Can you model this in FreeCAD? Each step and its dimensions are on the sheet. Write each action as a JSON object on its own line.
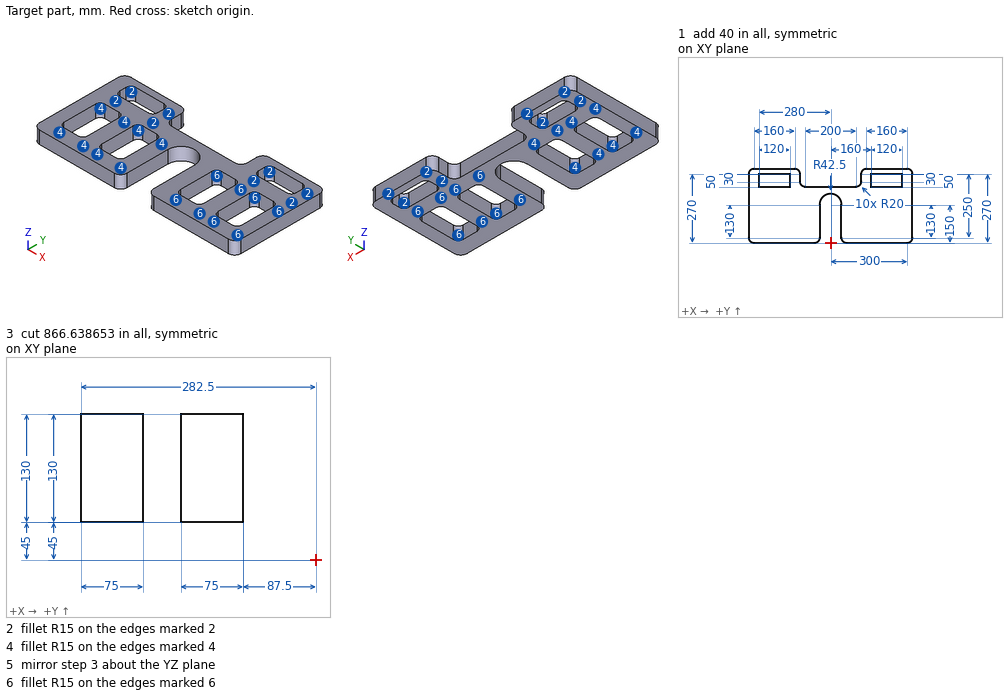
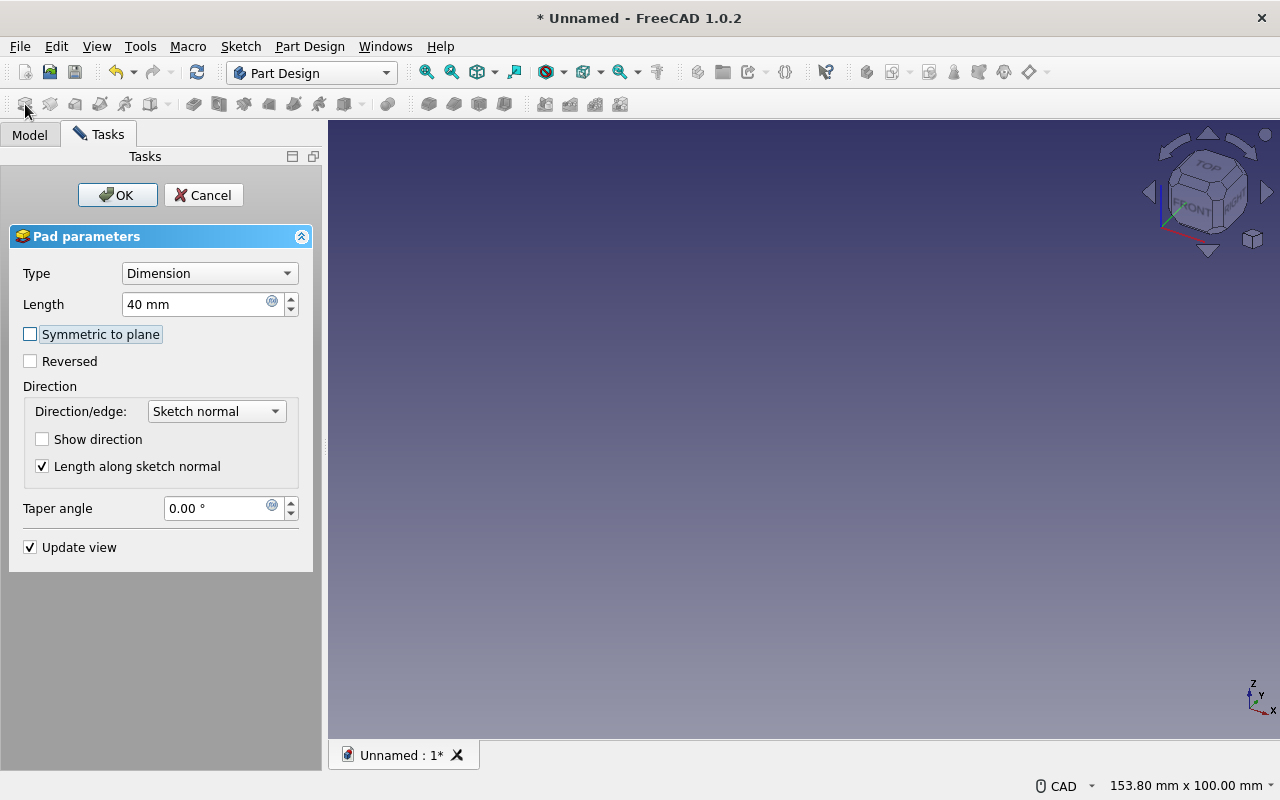
{"action": "left_click", "coordinate": [31, 334]}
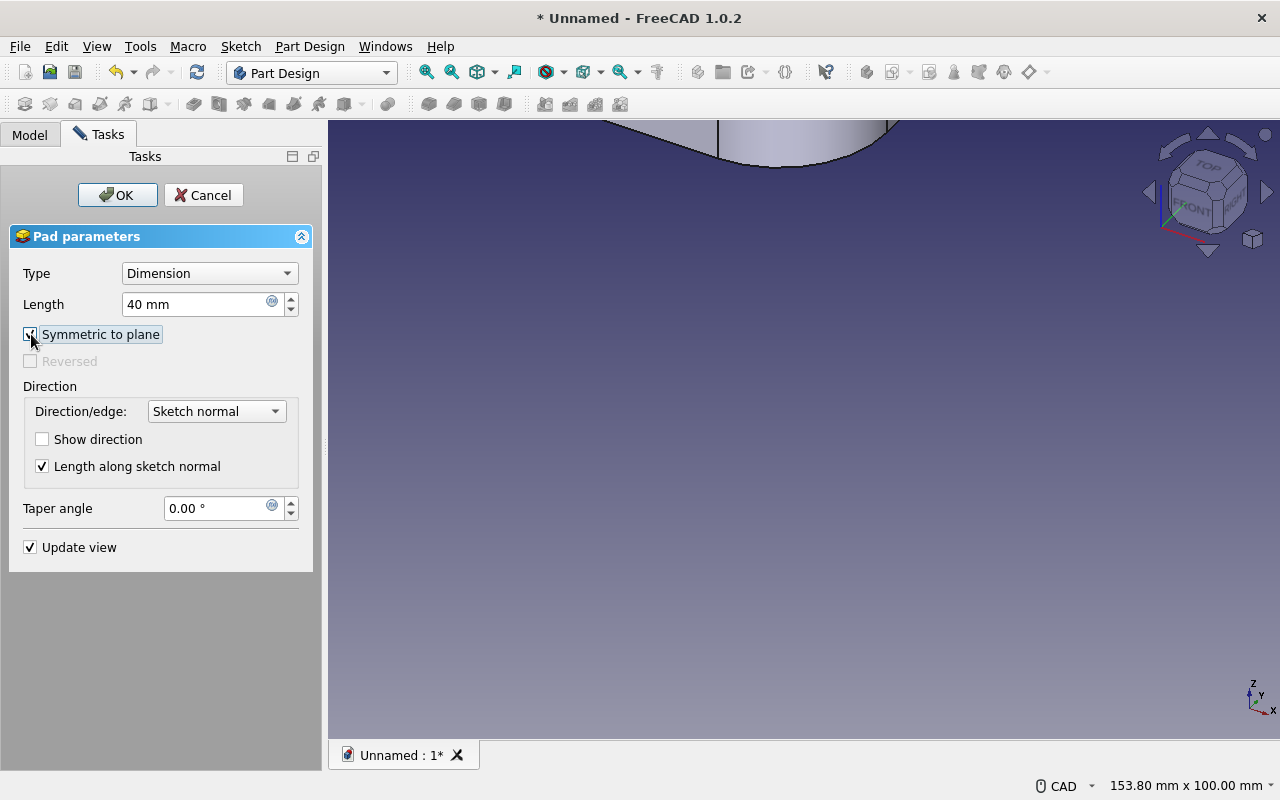
{"action": "left_click", "coordinate": [118, 195]}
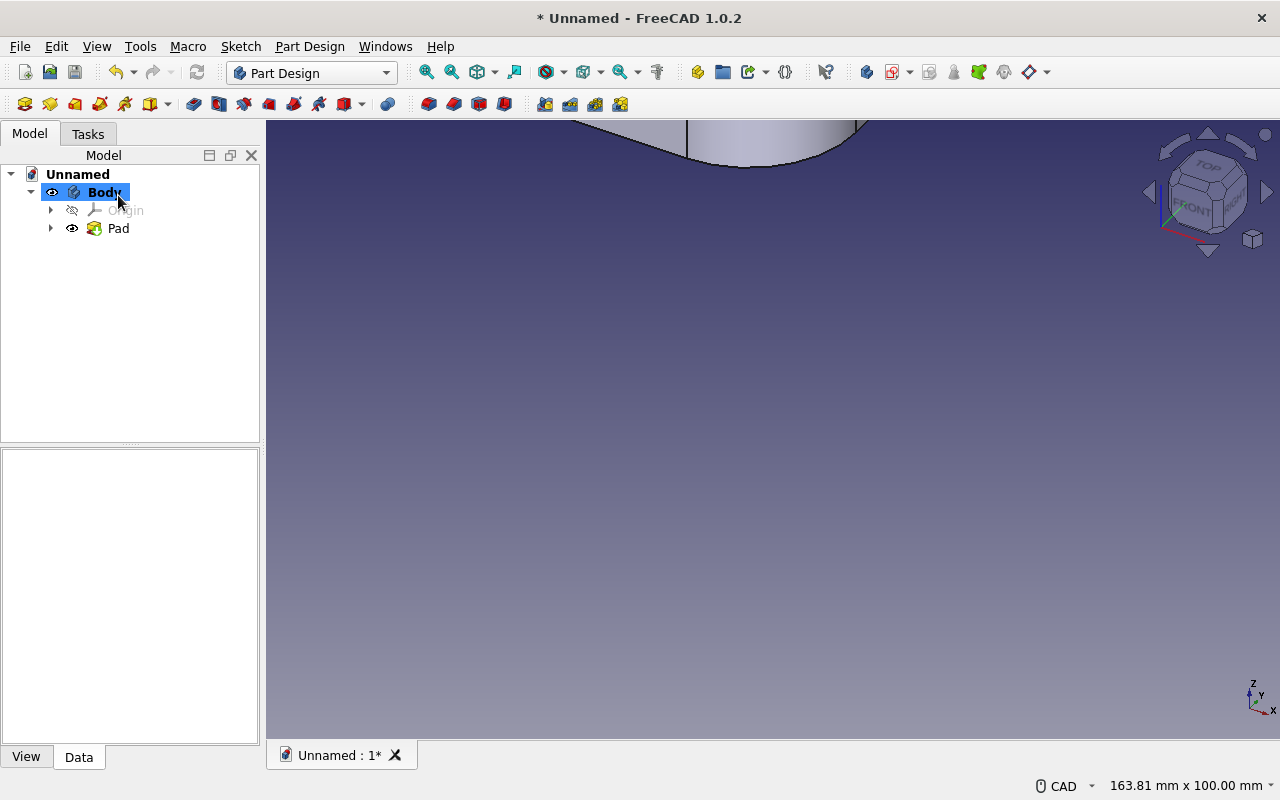
{"action": "key", "text": "v f"}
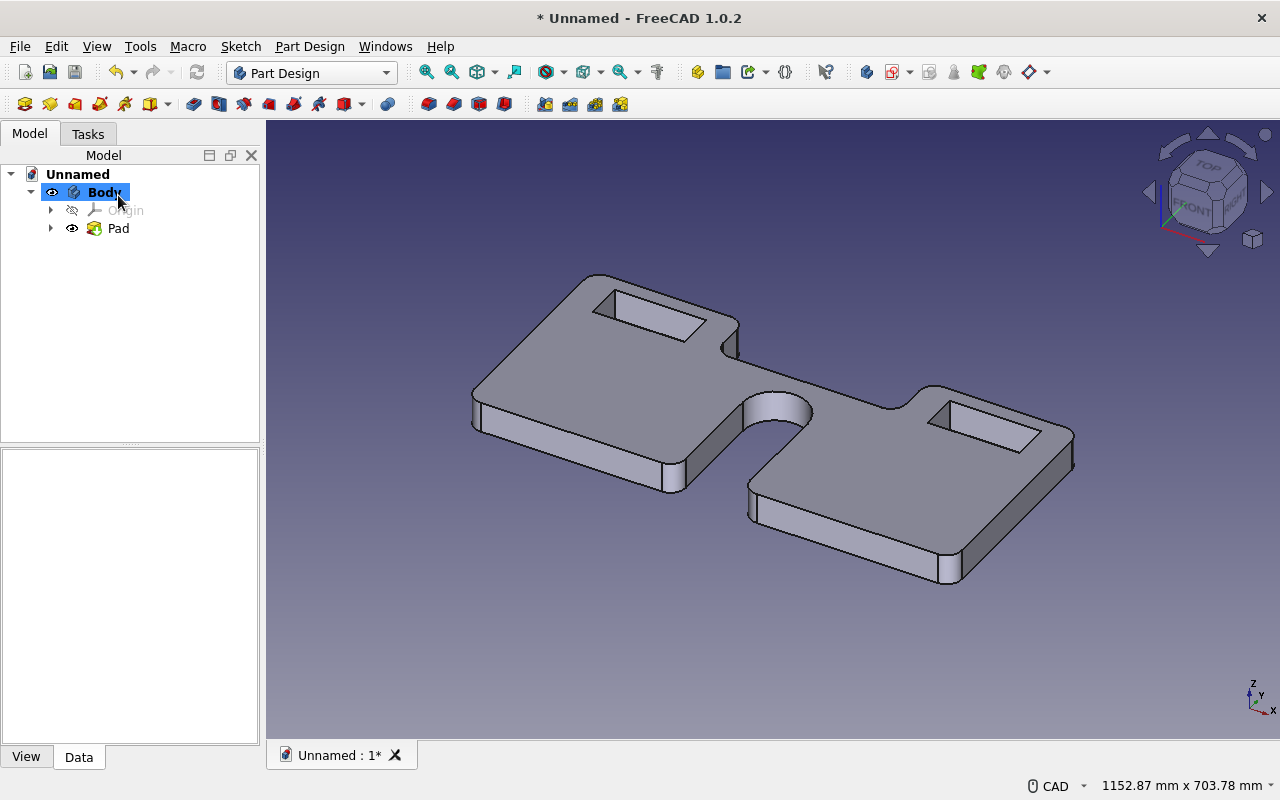
{"action": "key", "text": "0"}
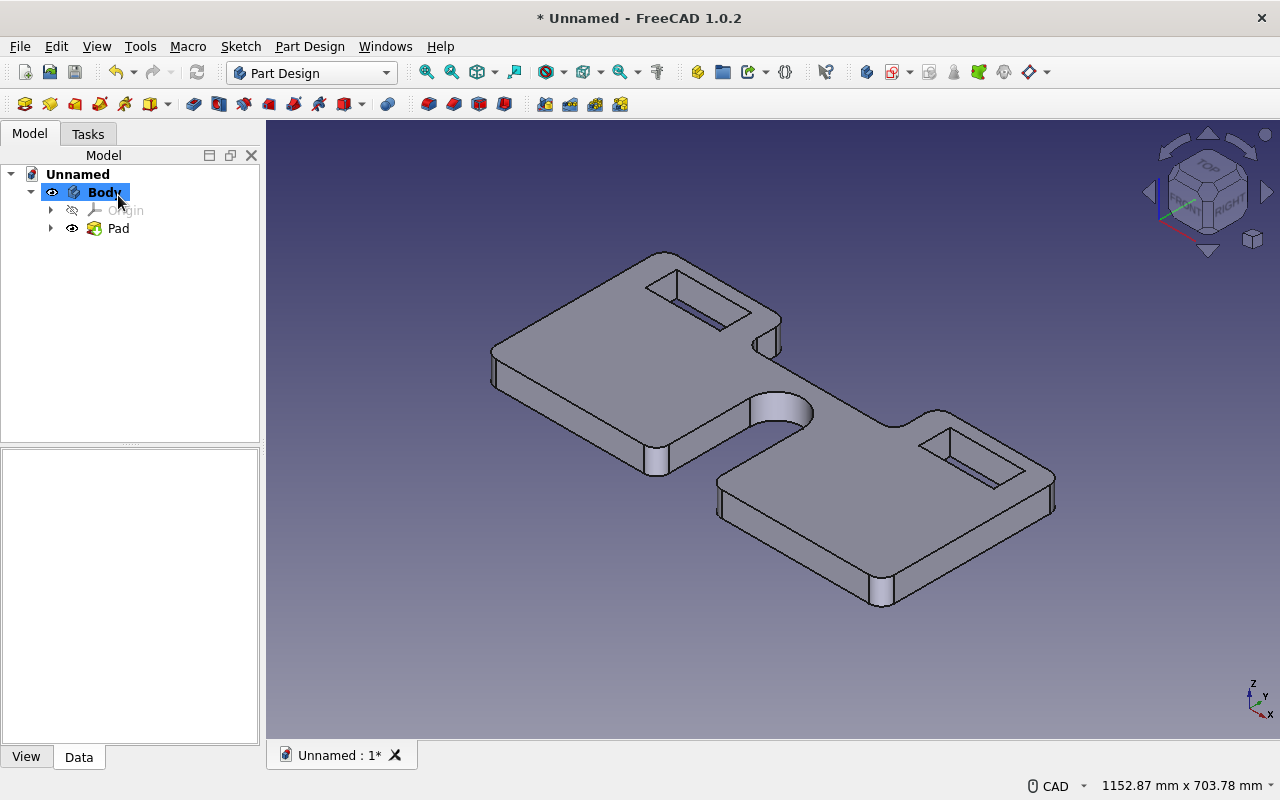
{"action": "key", "text": "2"}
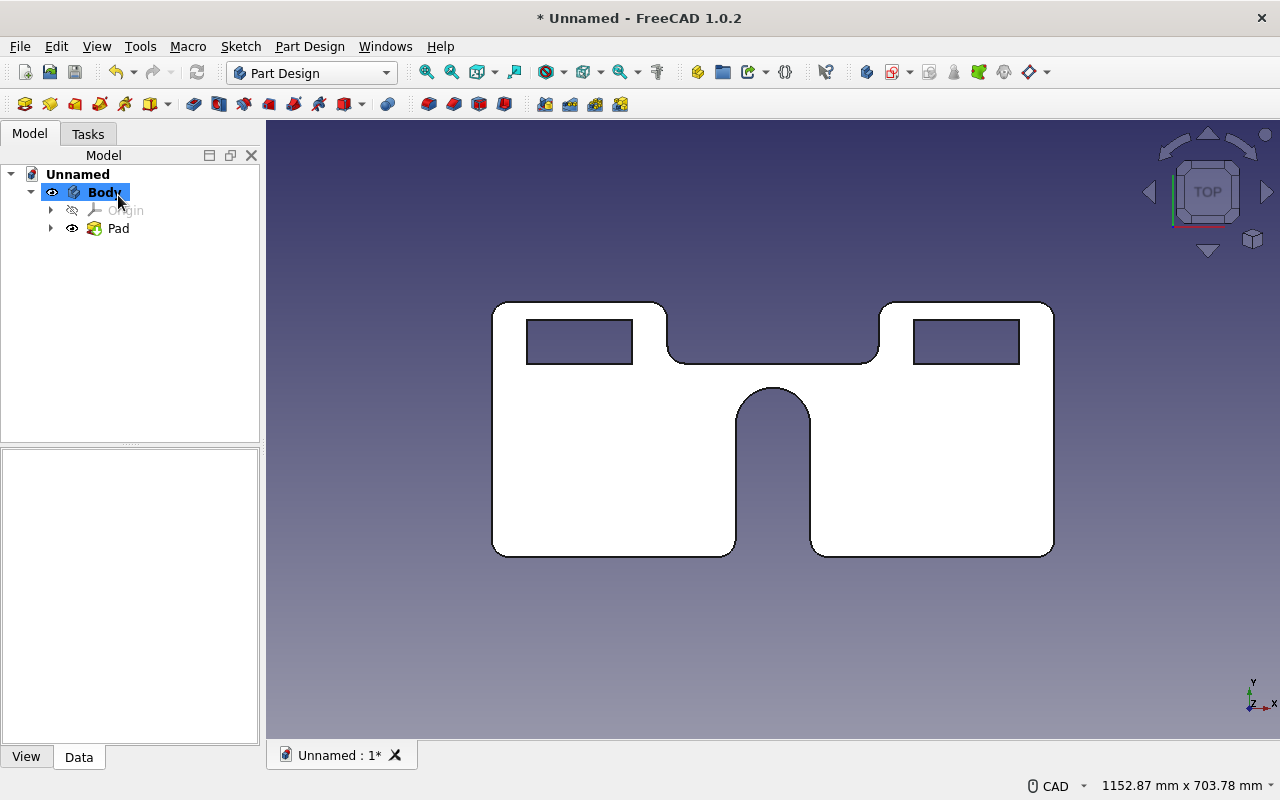
{"action": "key", "text": "1"}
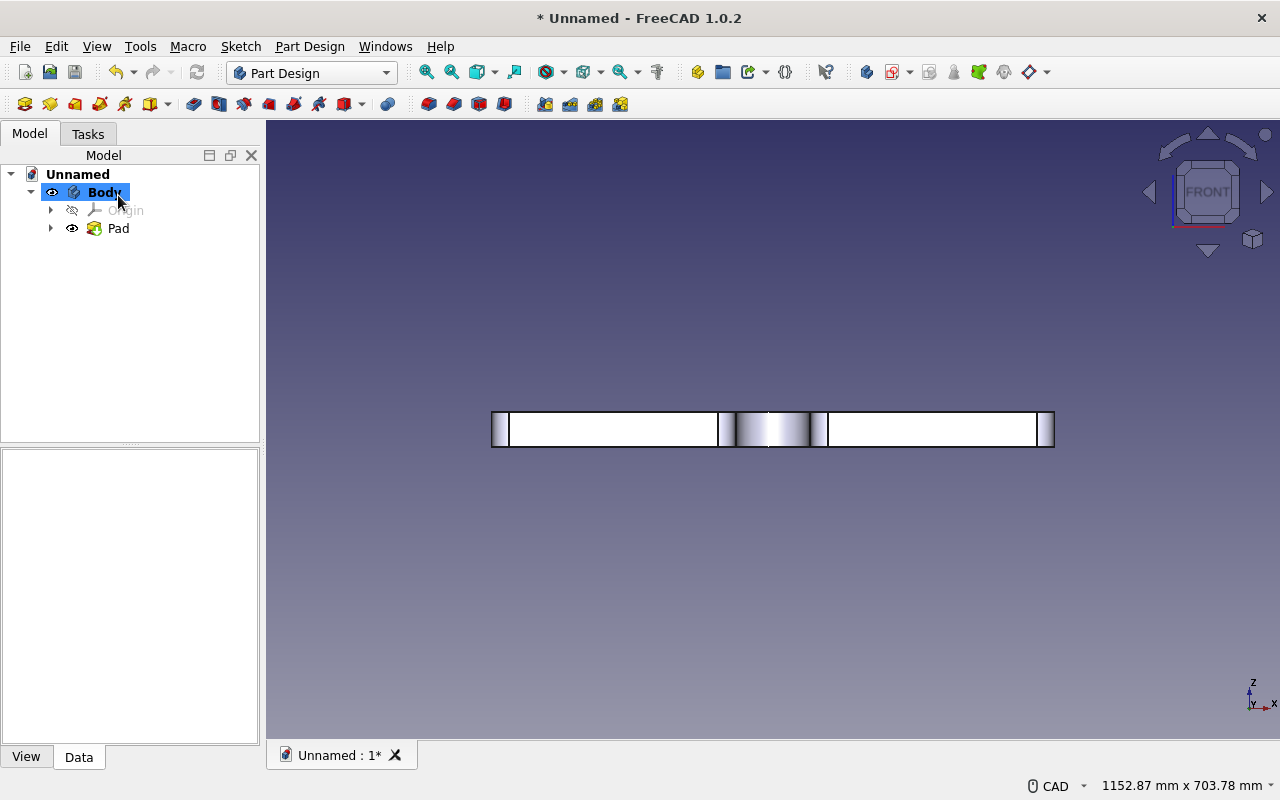
{"action": "key", "text": "3"}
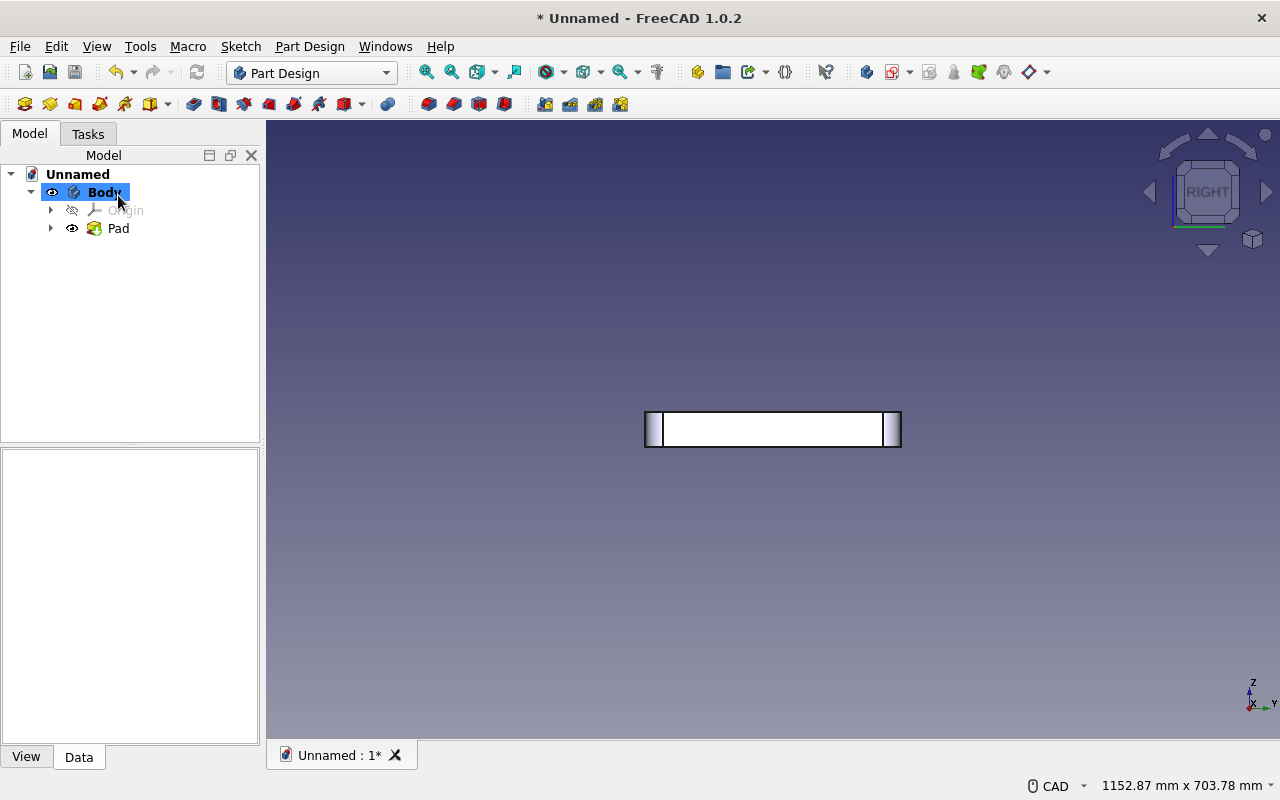
{"action": "key", "text": "v f"}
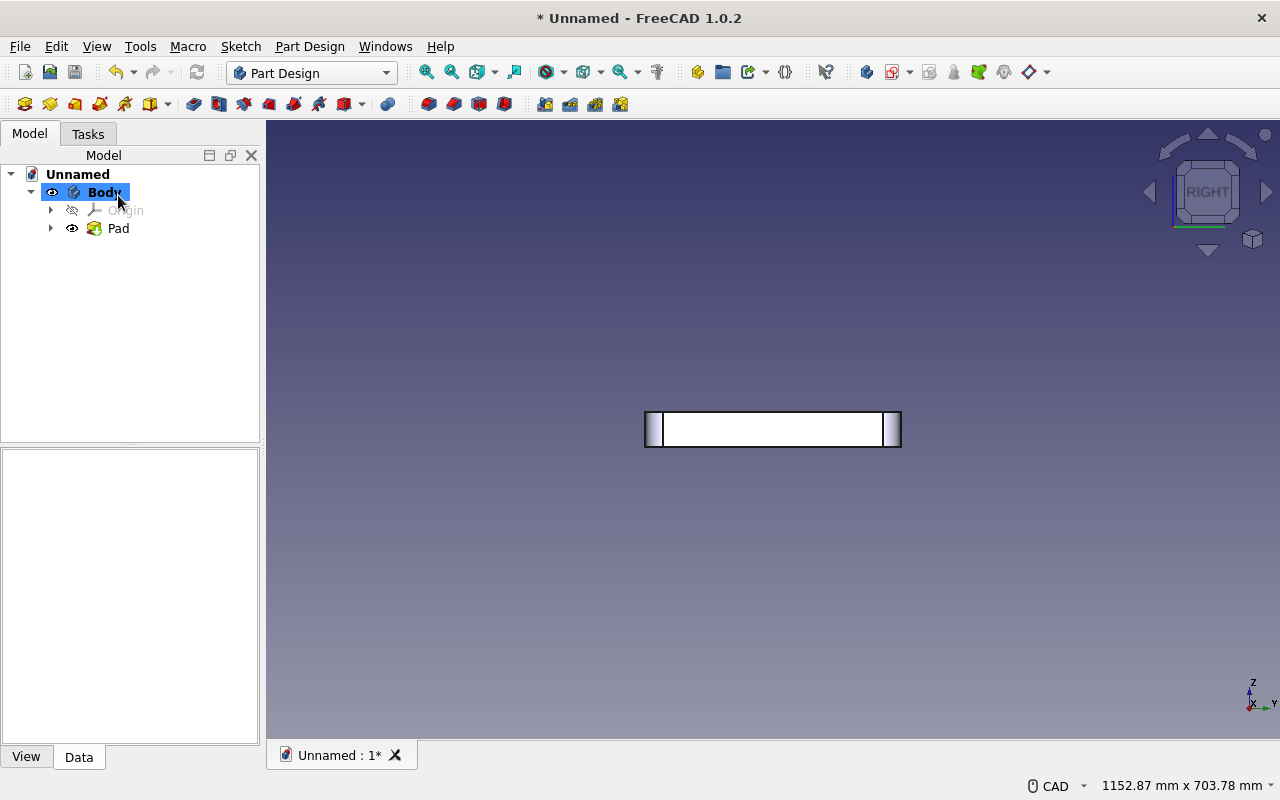
{"action": "key", "text": "5"}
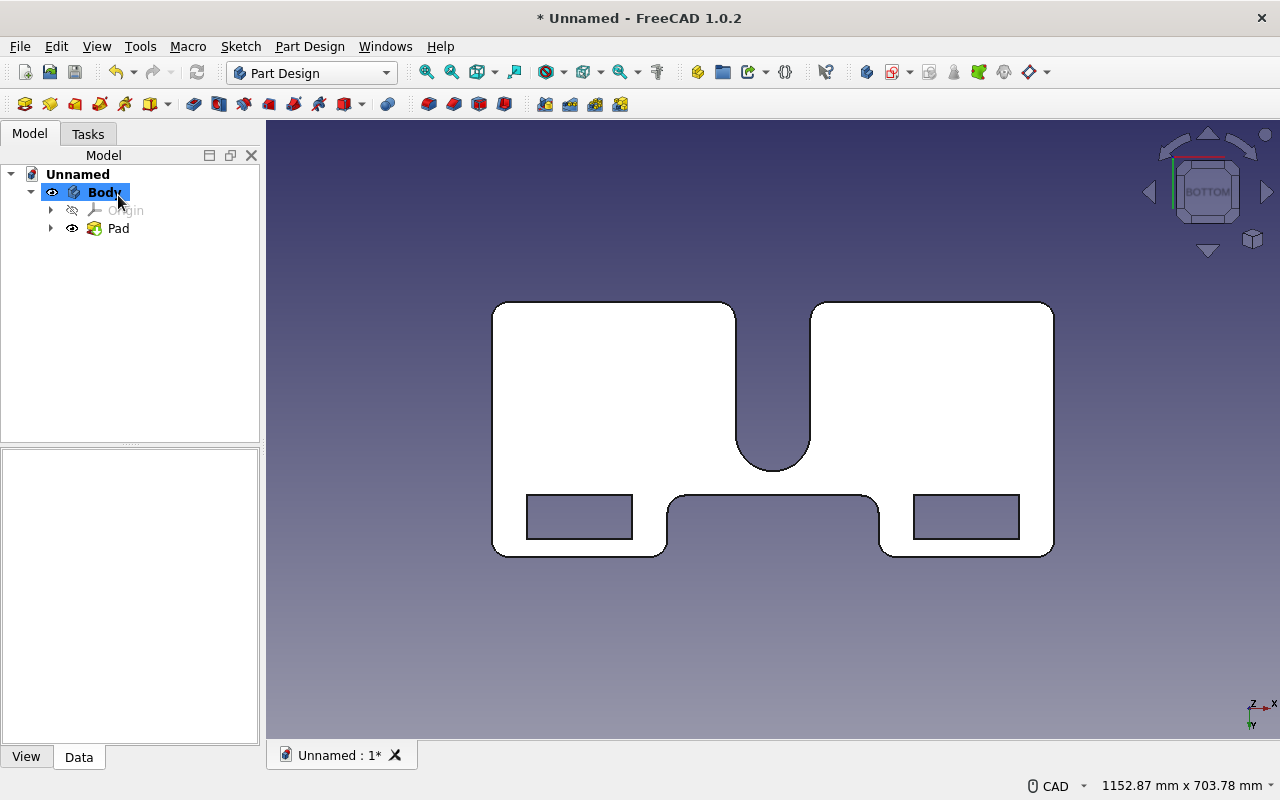
{"action": "key", "text": "4"}